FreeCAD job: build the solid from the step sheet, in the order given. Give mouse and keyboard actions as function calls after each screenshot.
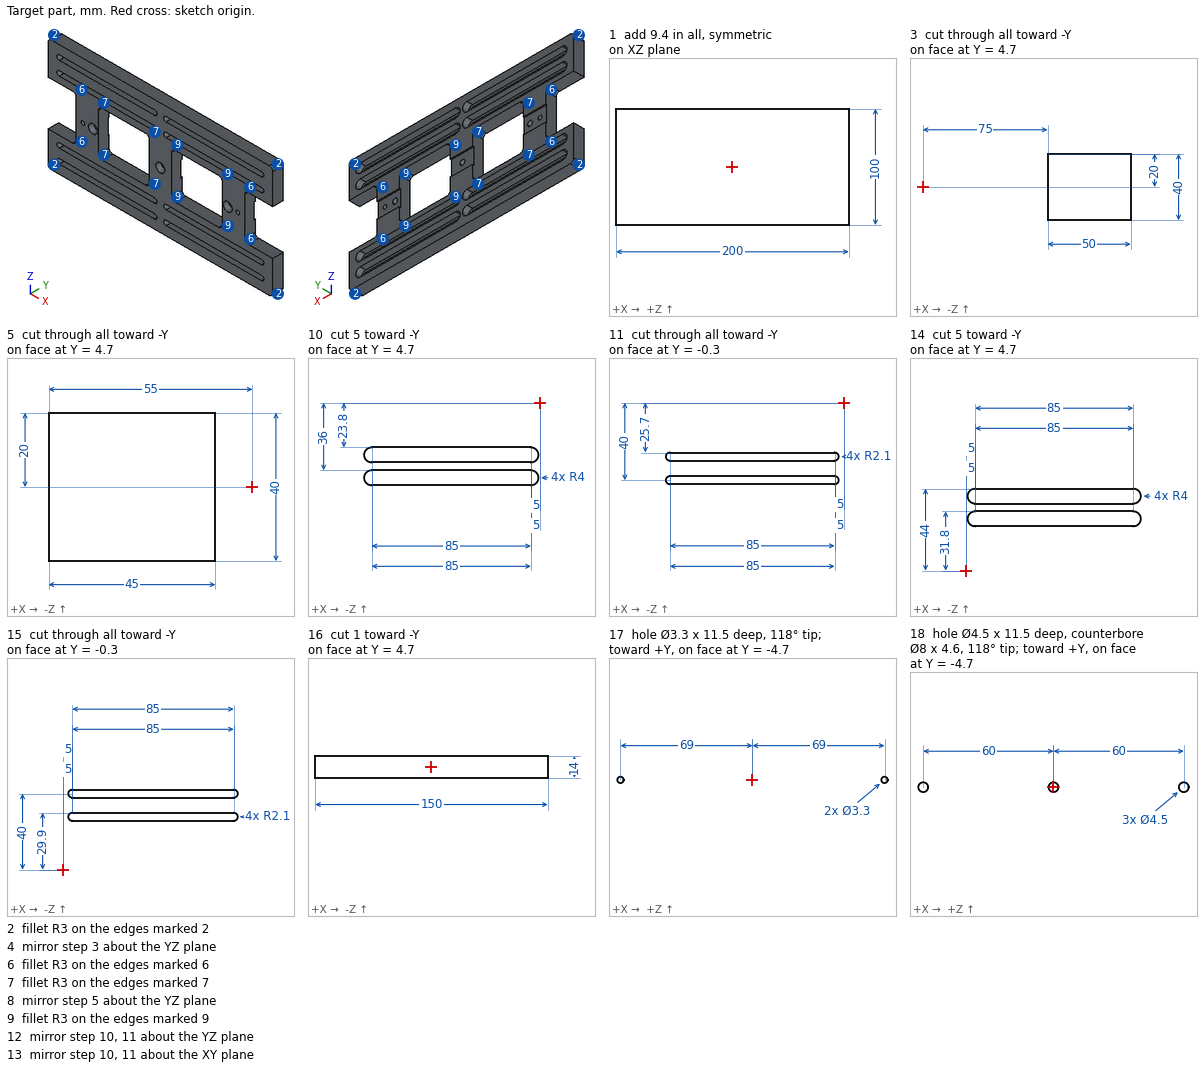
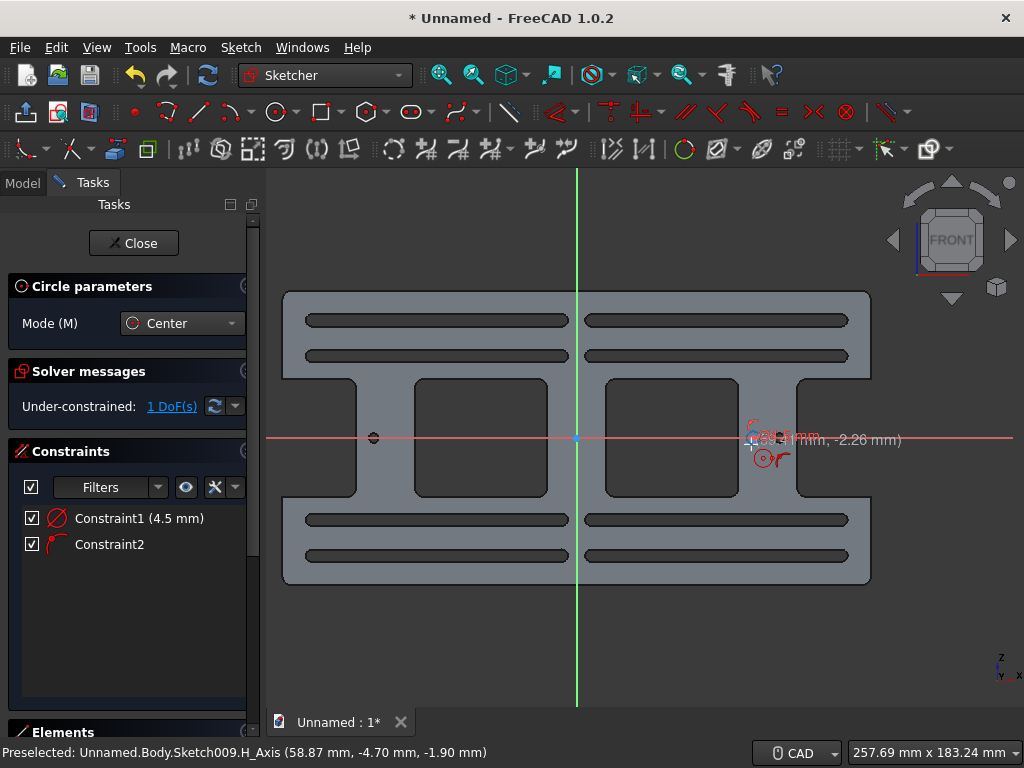
scroll(577, 438, up, 7)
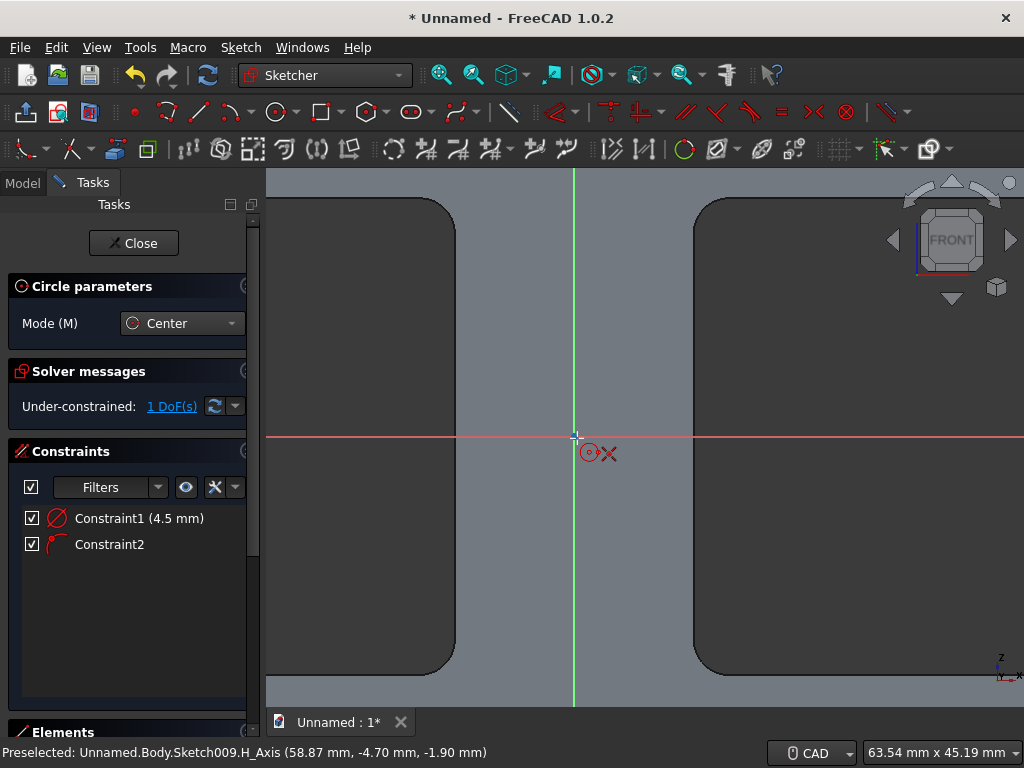
scroll(577, 438, down, 7)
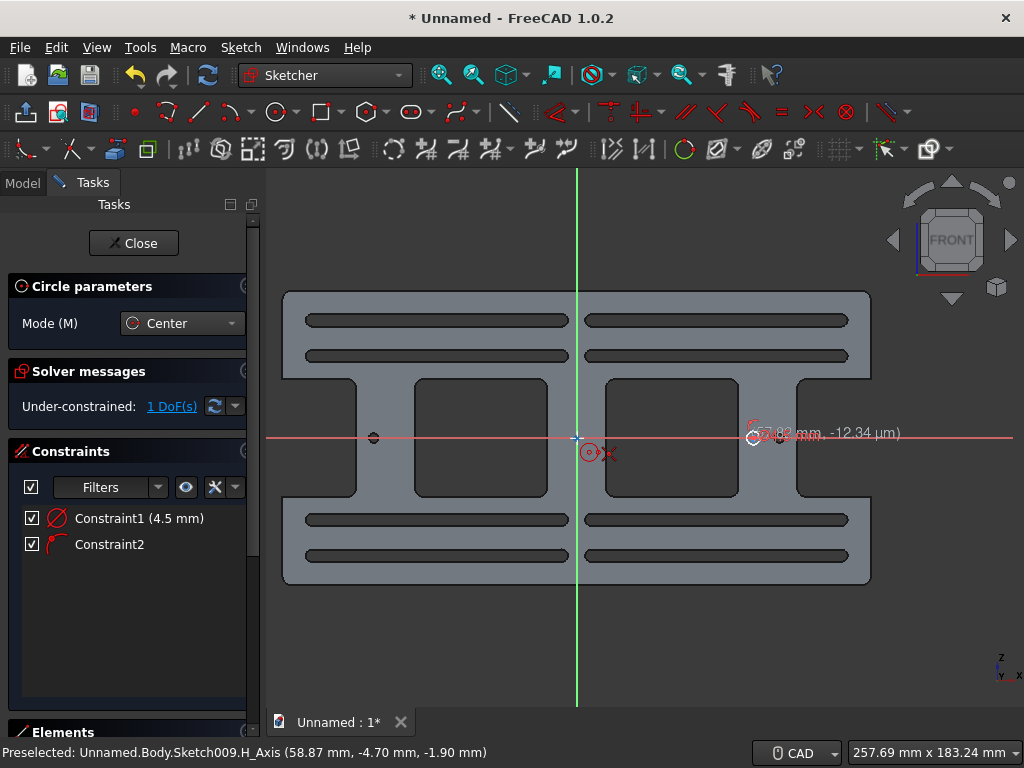
click(577, 438)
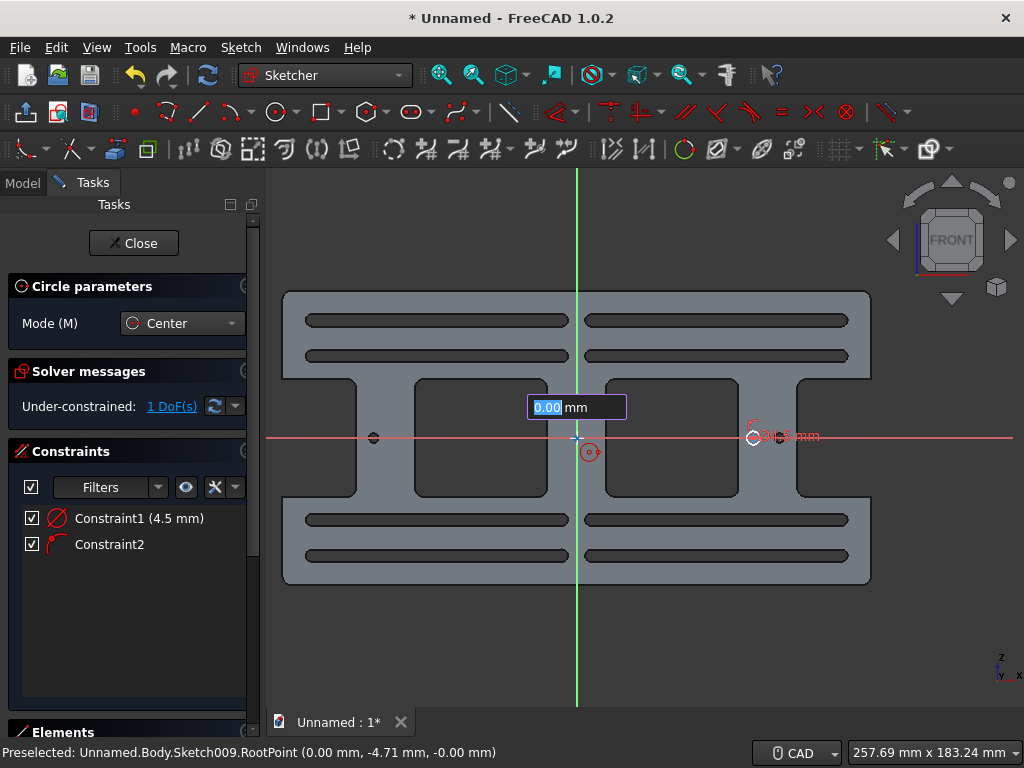
scroll(581, 433, up, 7)
move(581, 433)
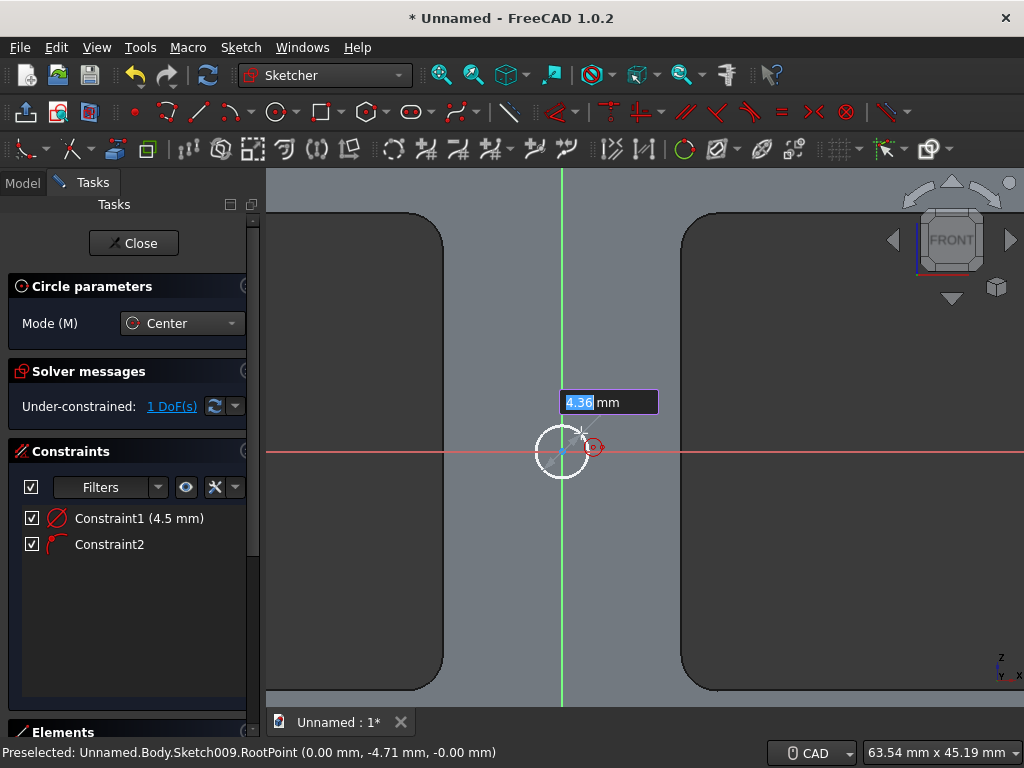
text(4.5)
key(Return)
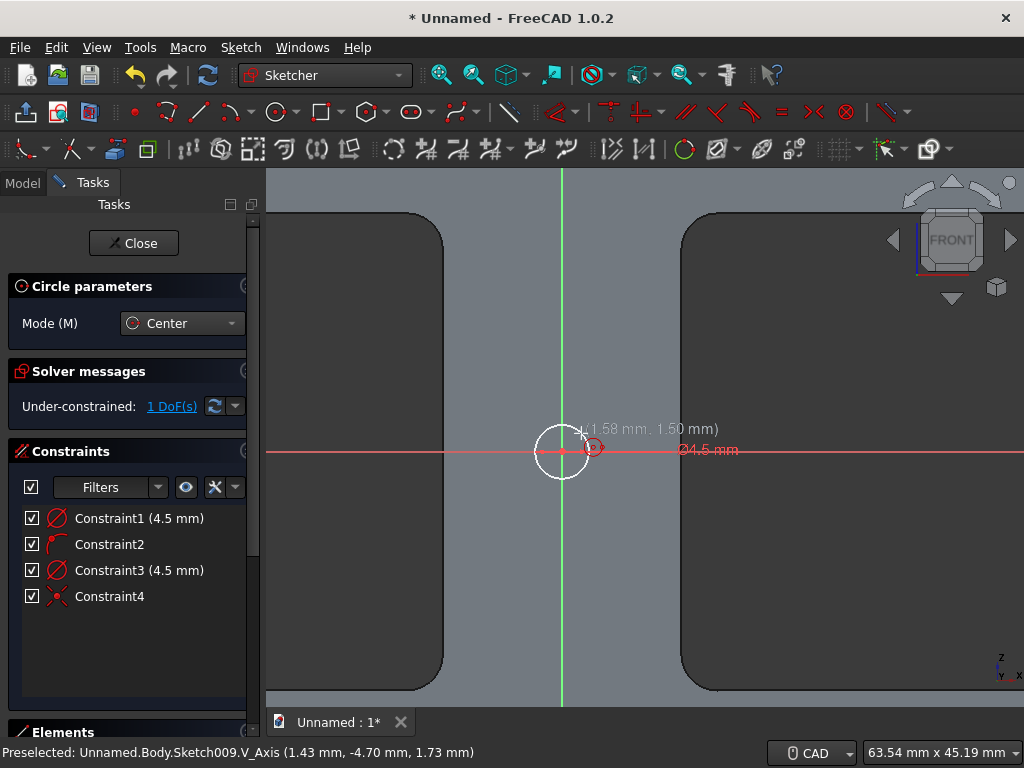
scroll(581, 433, down, 7)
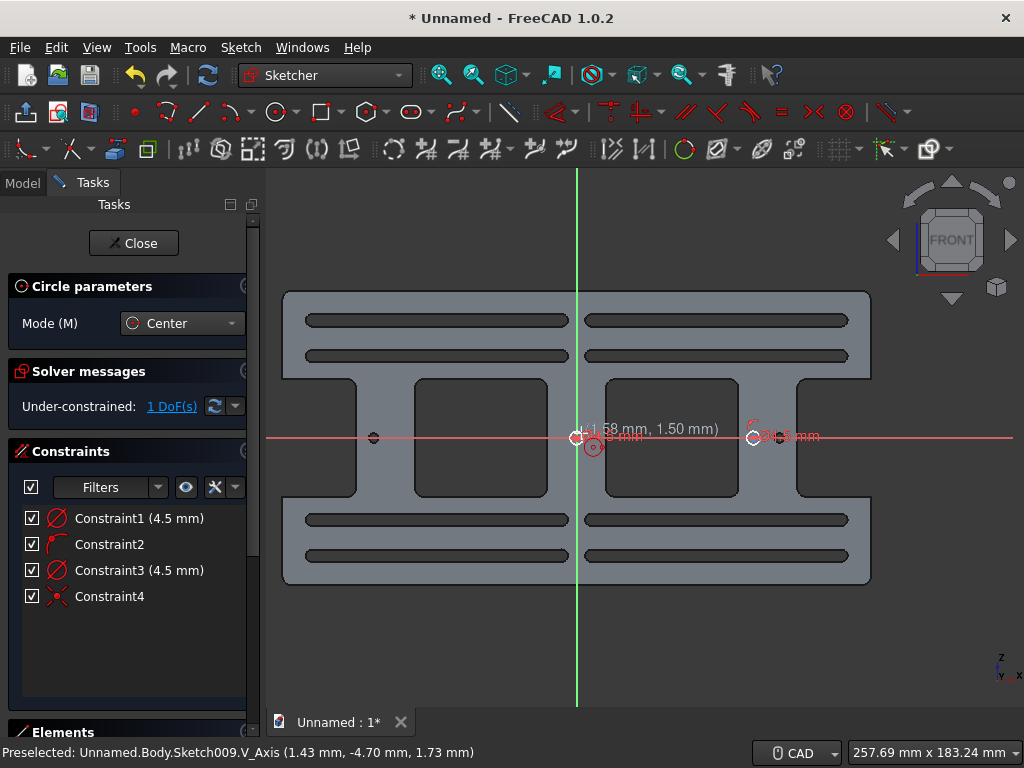
scroll(400, 438, up, 7)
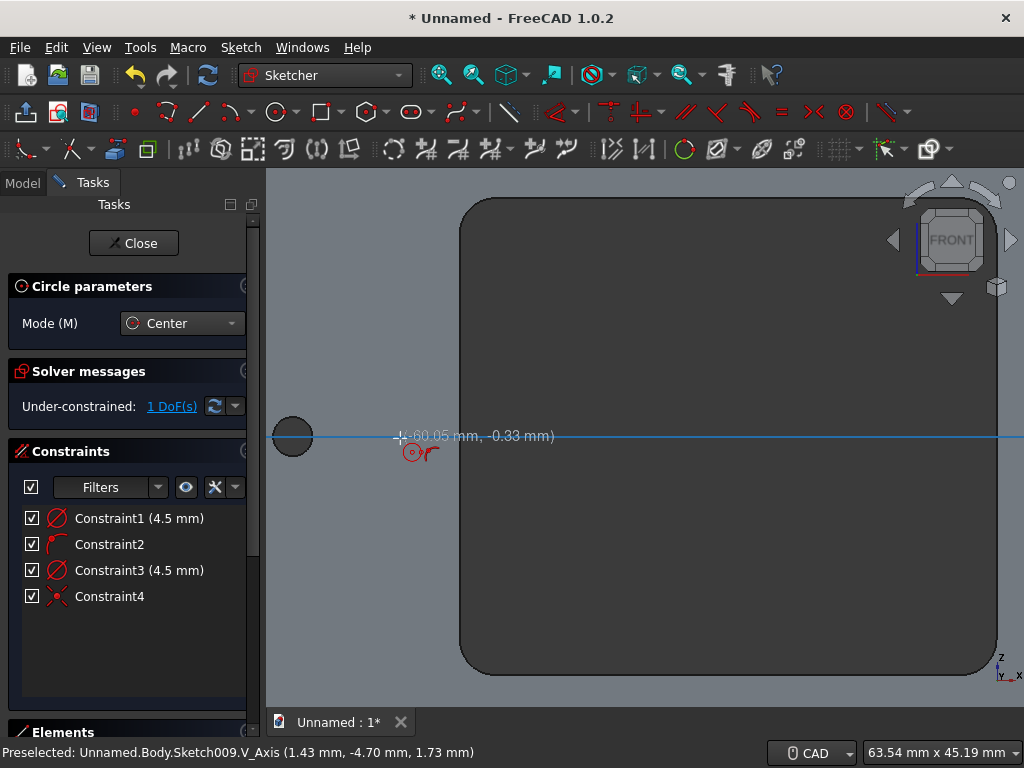
scroll(400, 438, down, 7)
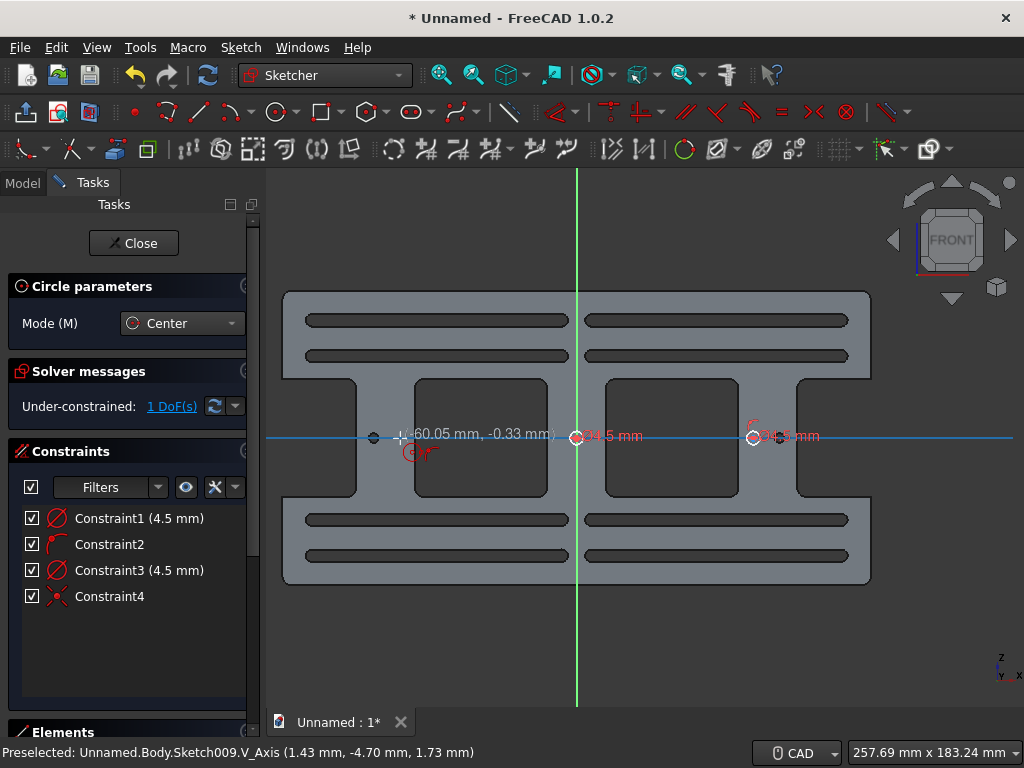
click(400, 438)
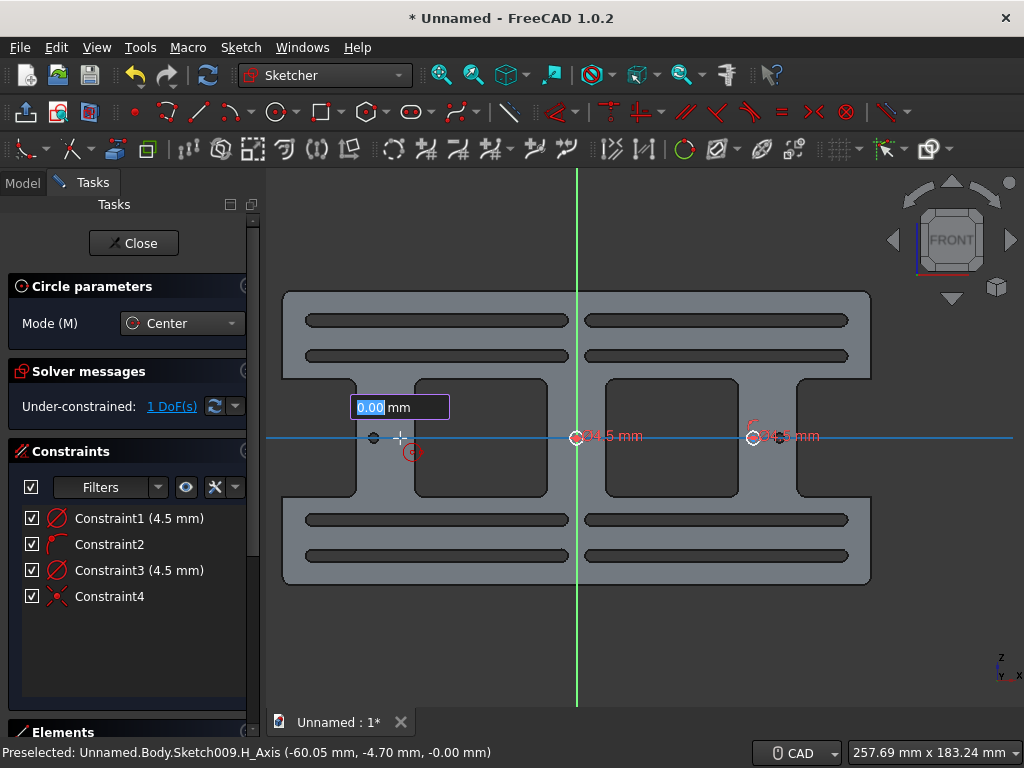
scroll(398, 444, up, 5)
move(397, 444)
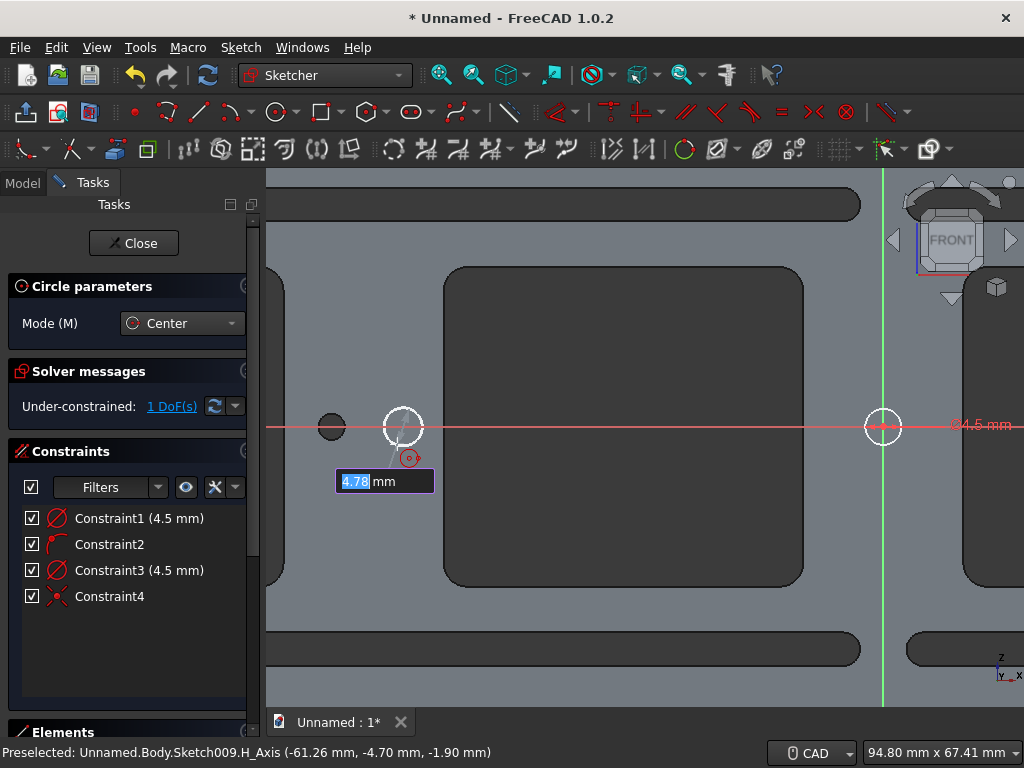
text(4.5)
key(Return)
key(Escape)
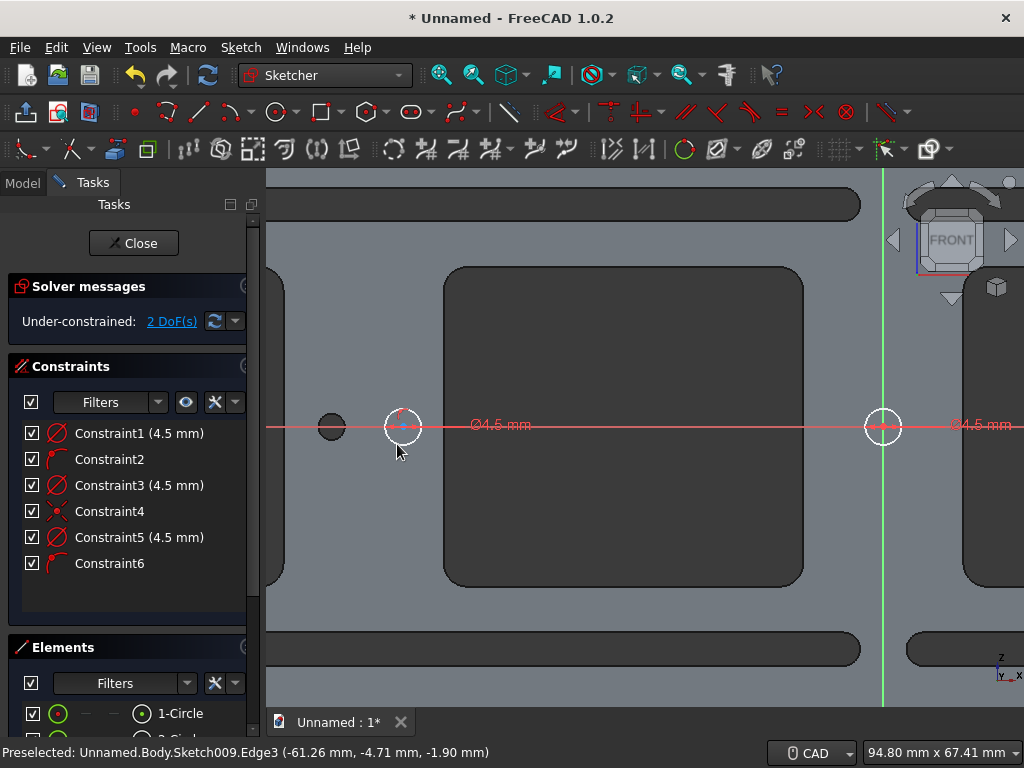
key(d)